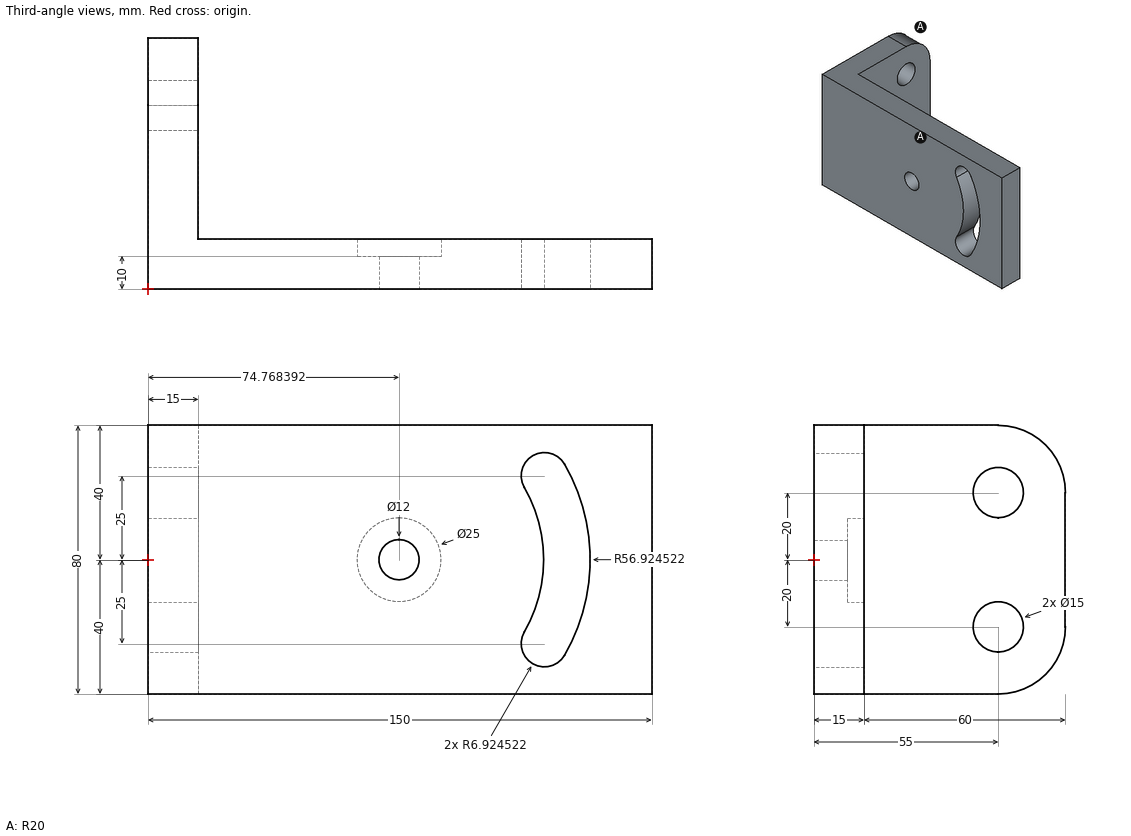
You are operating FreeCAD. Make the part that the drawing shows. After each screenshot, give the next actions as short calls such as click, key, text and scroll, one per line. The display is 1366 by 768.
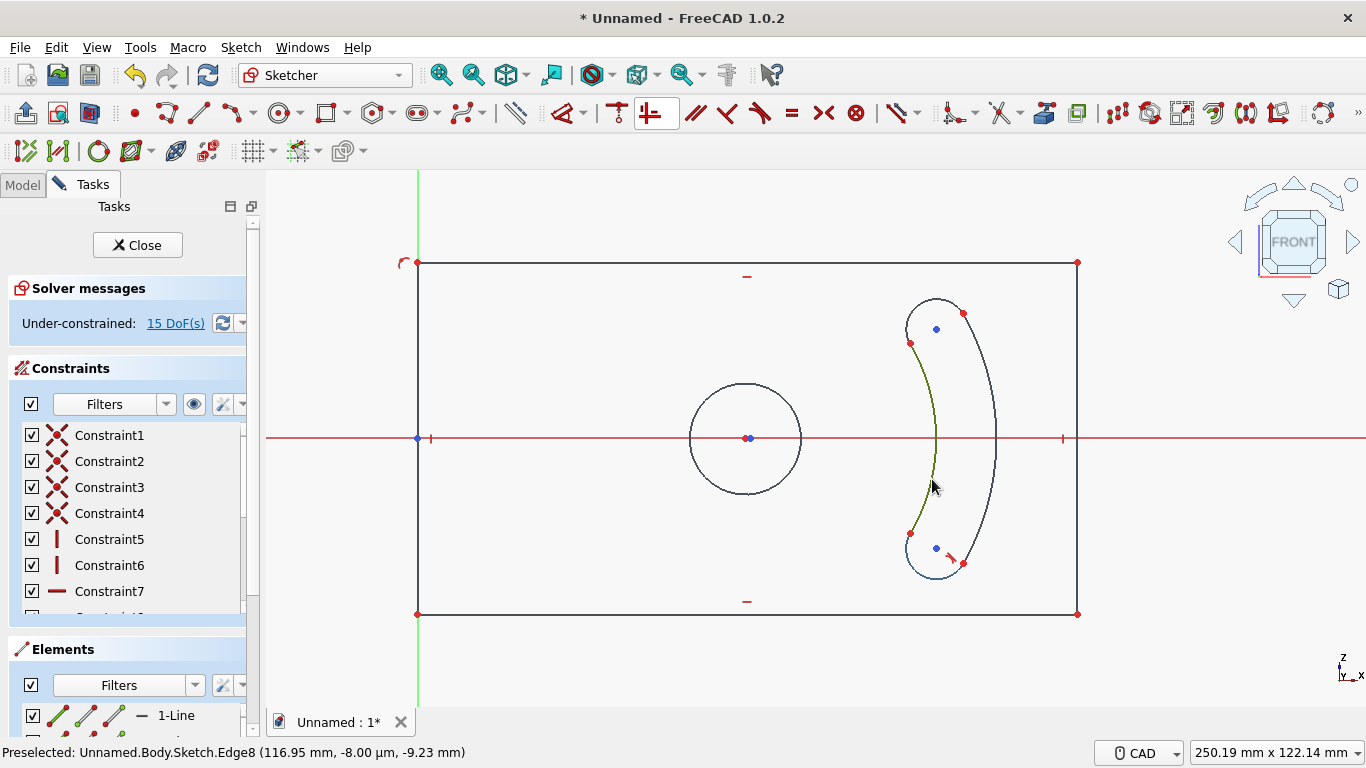
click(760, 114)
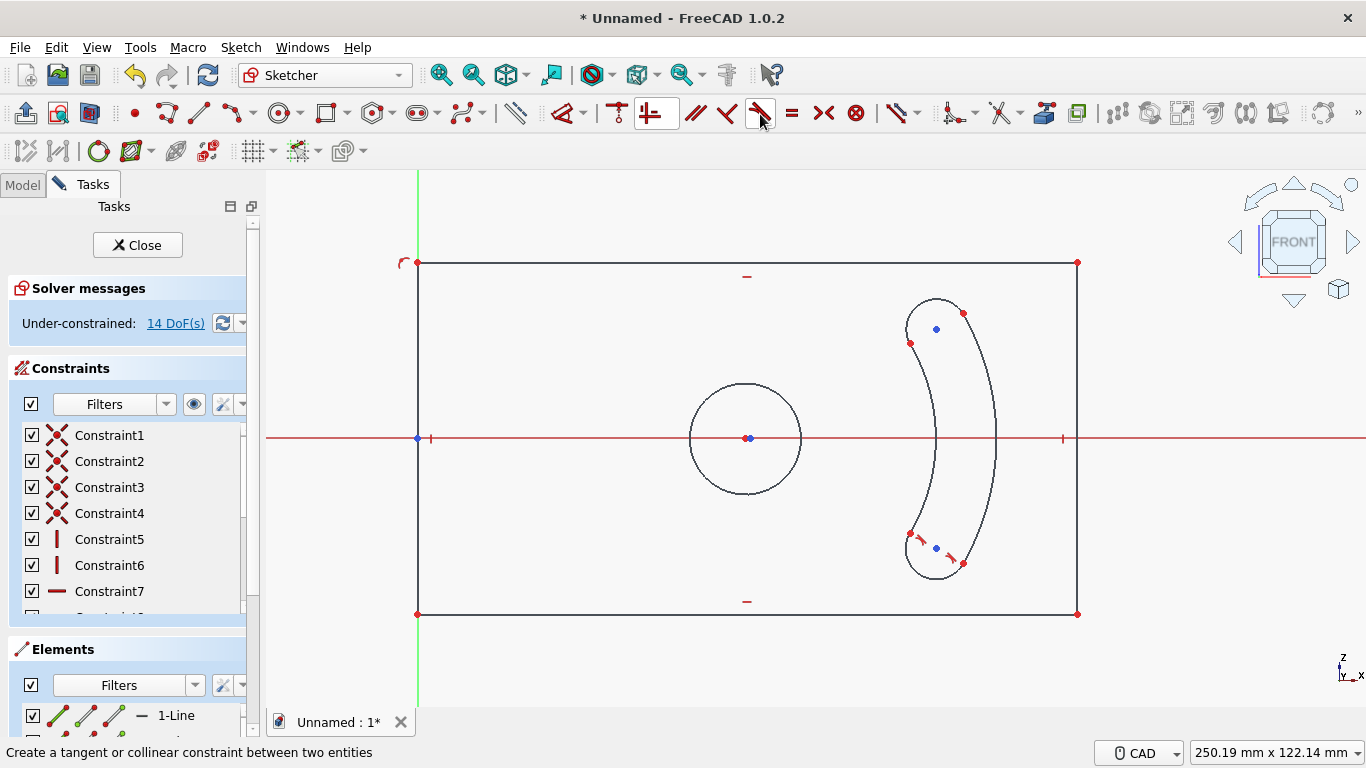
click(991, 491)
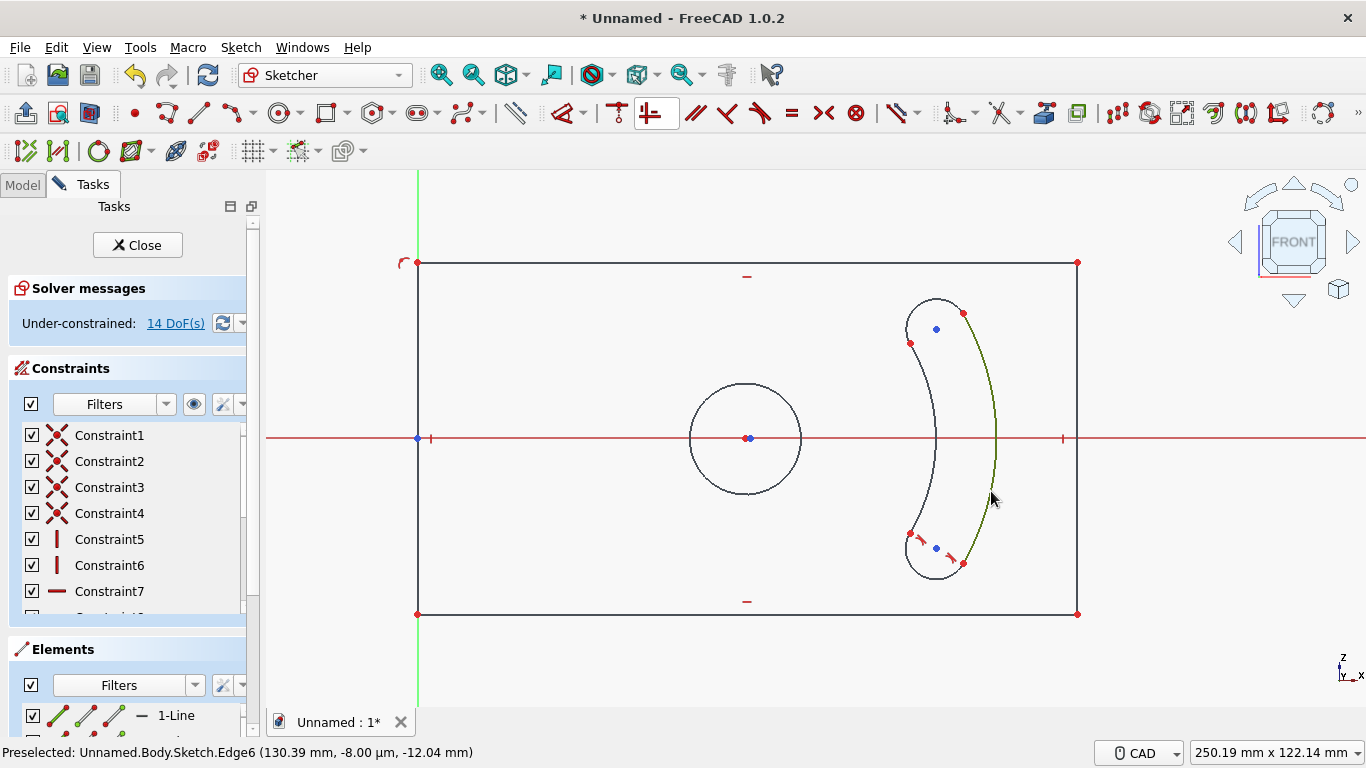
click(940, 299)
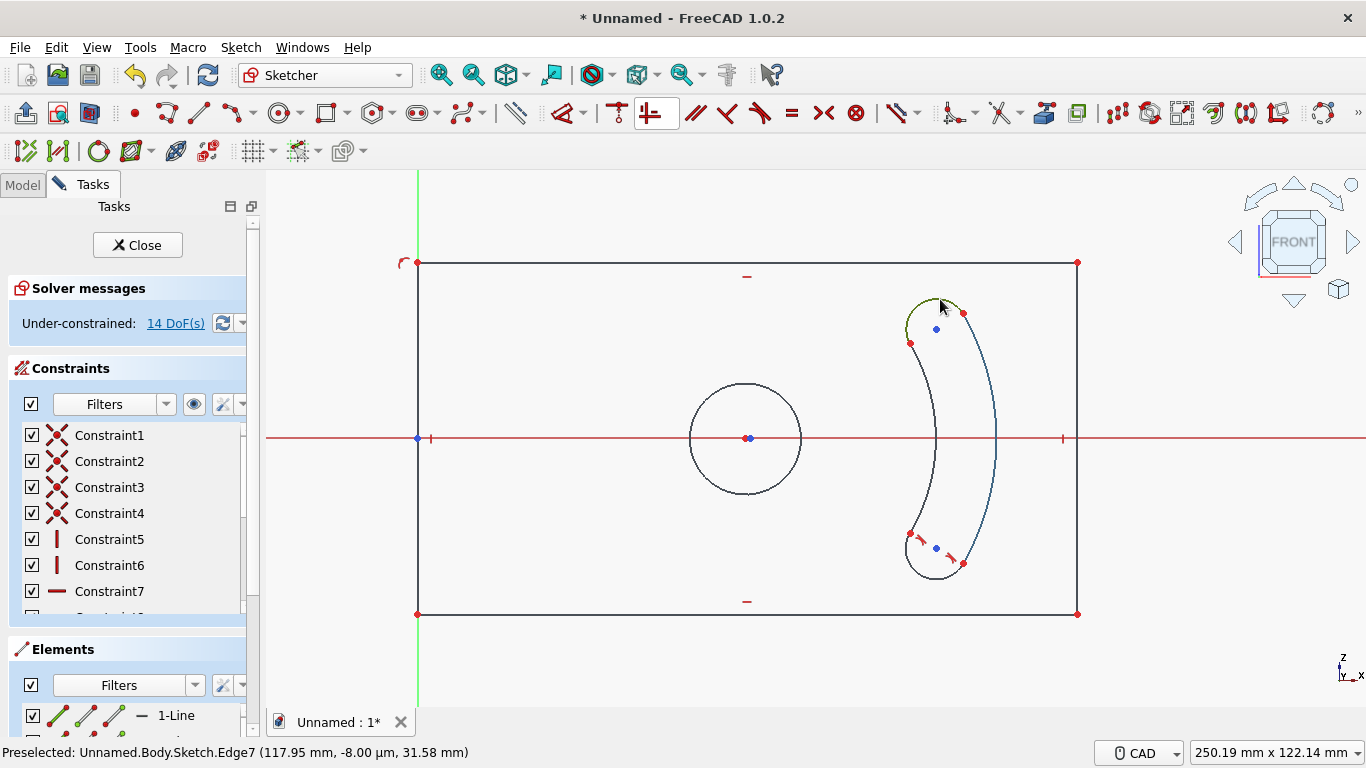
key(t)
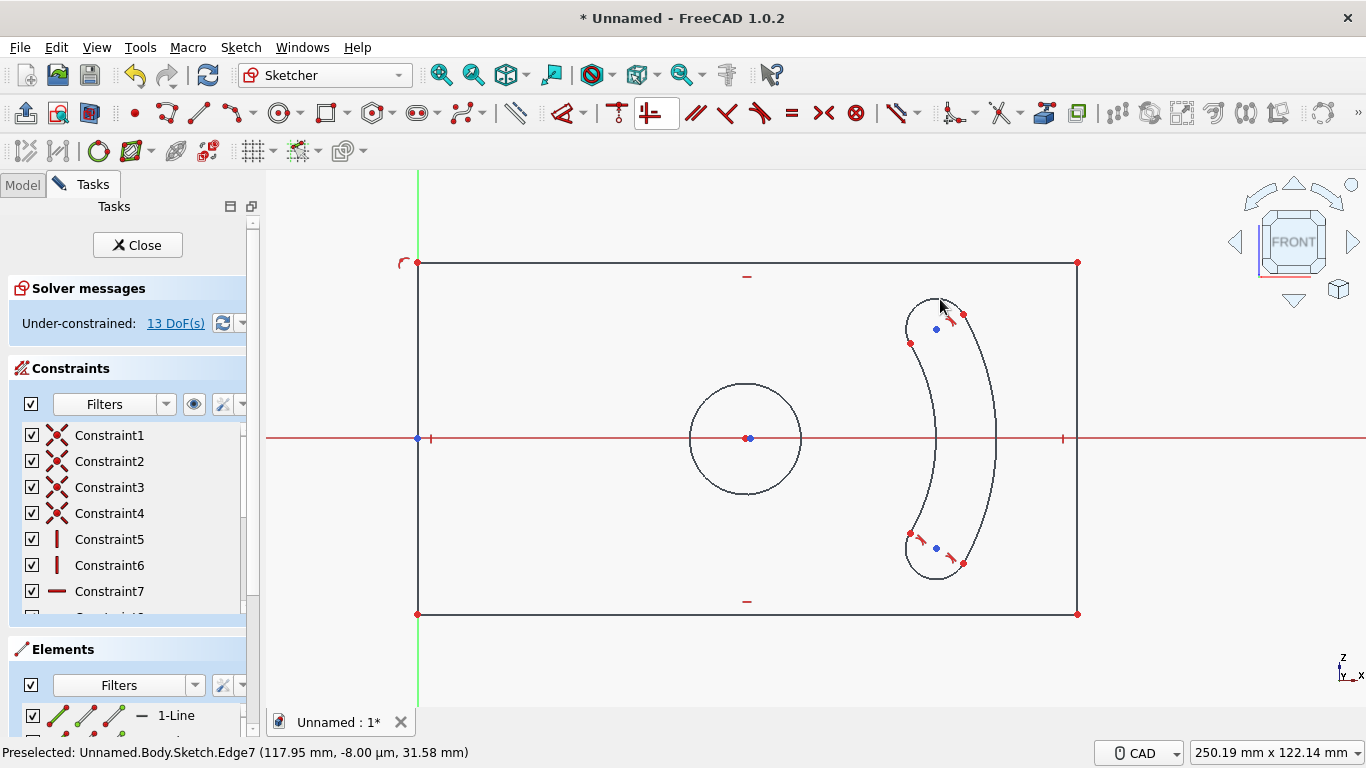
click(940, 299)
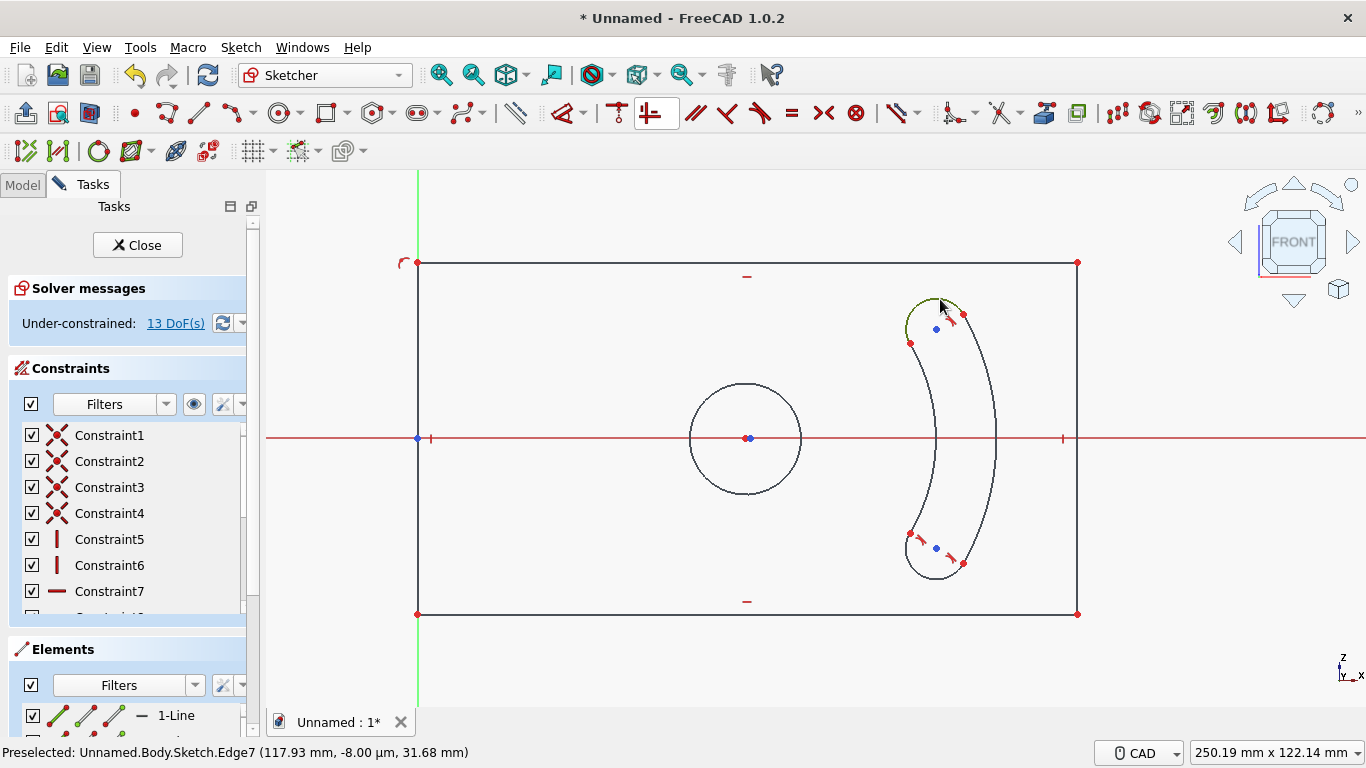
click(932, 478)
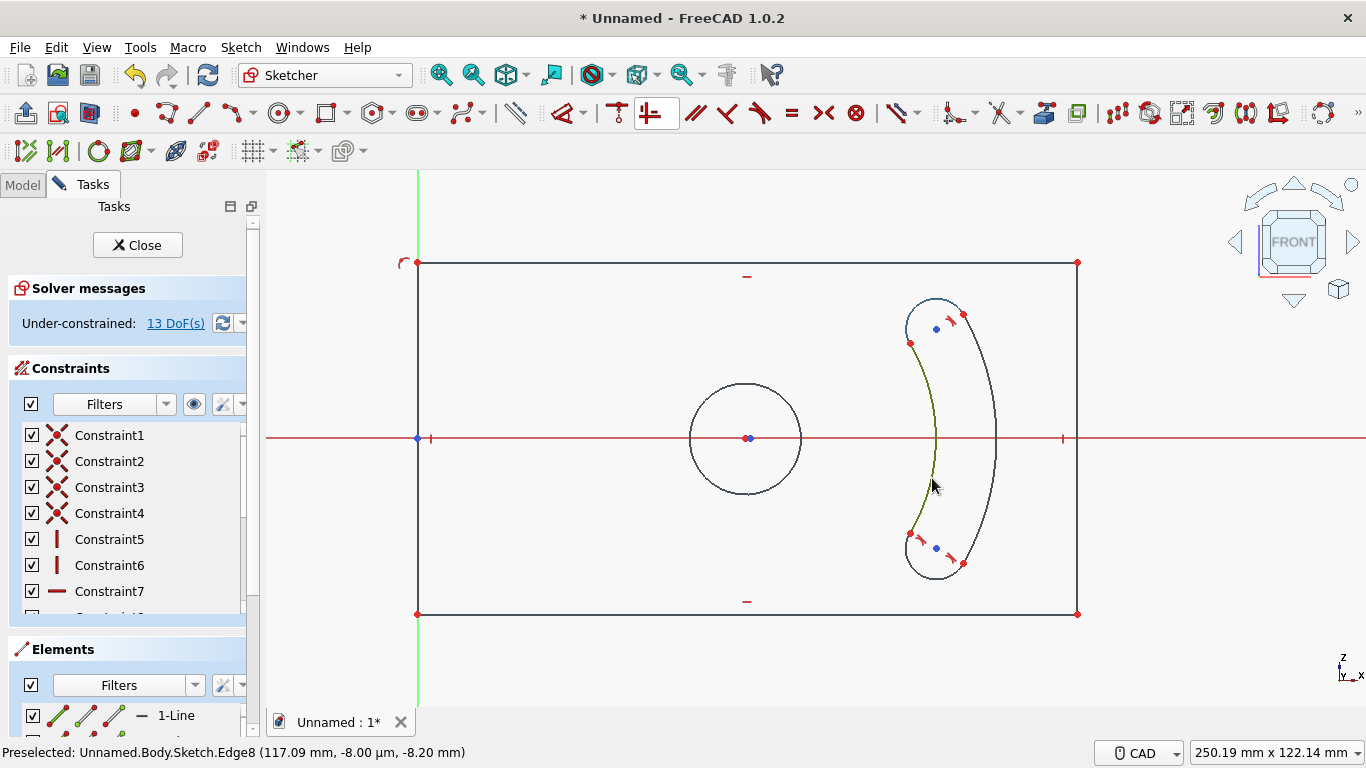
click(760, 114)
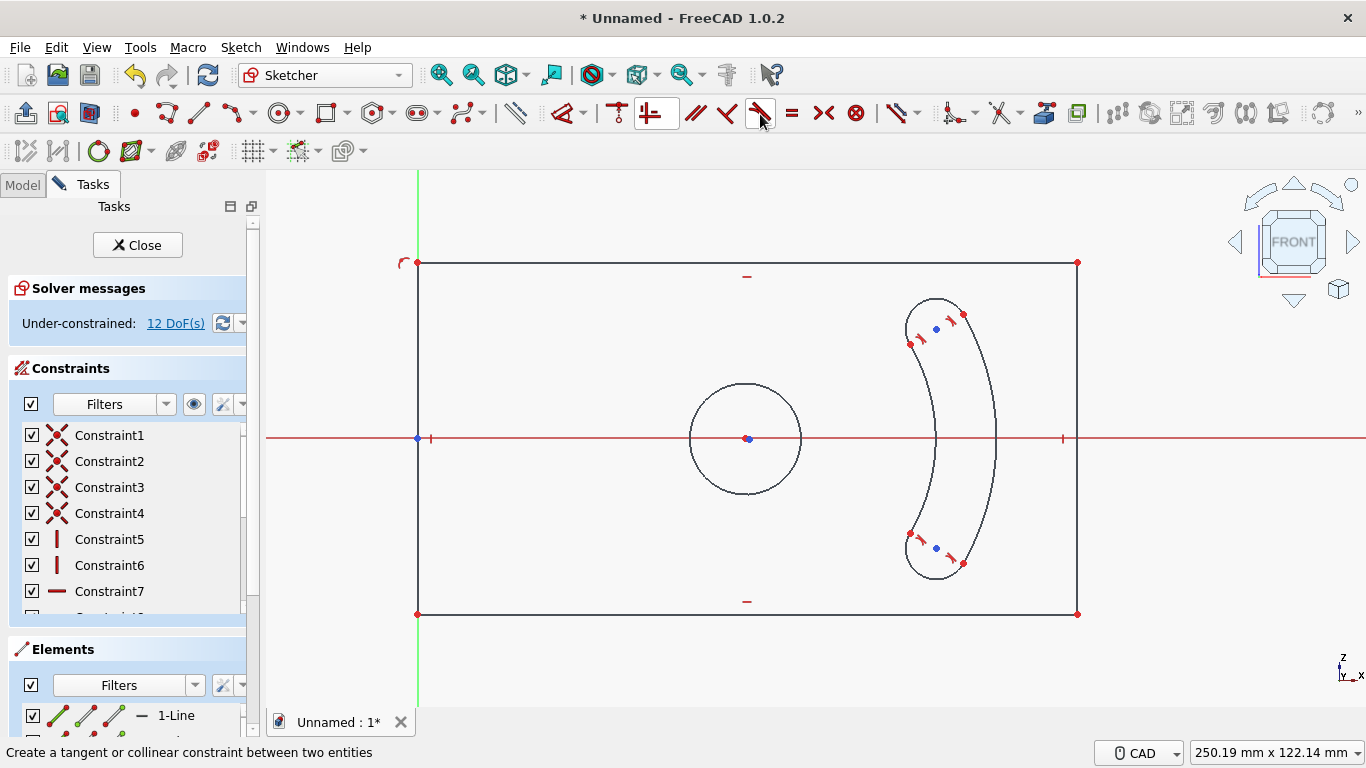
click(785, 400)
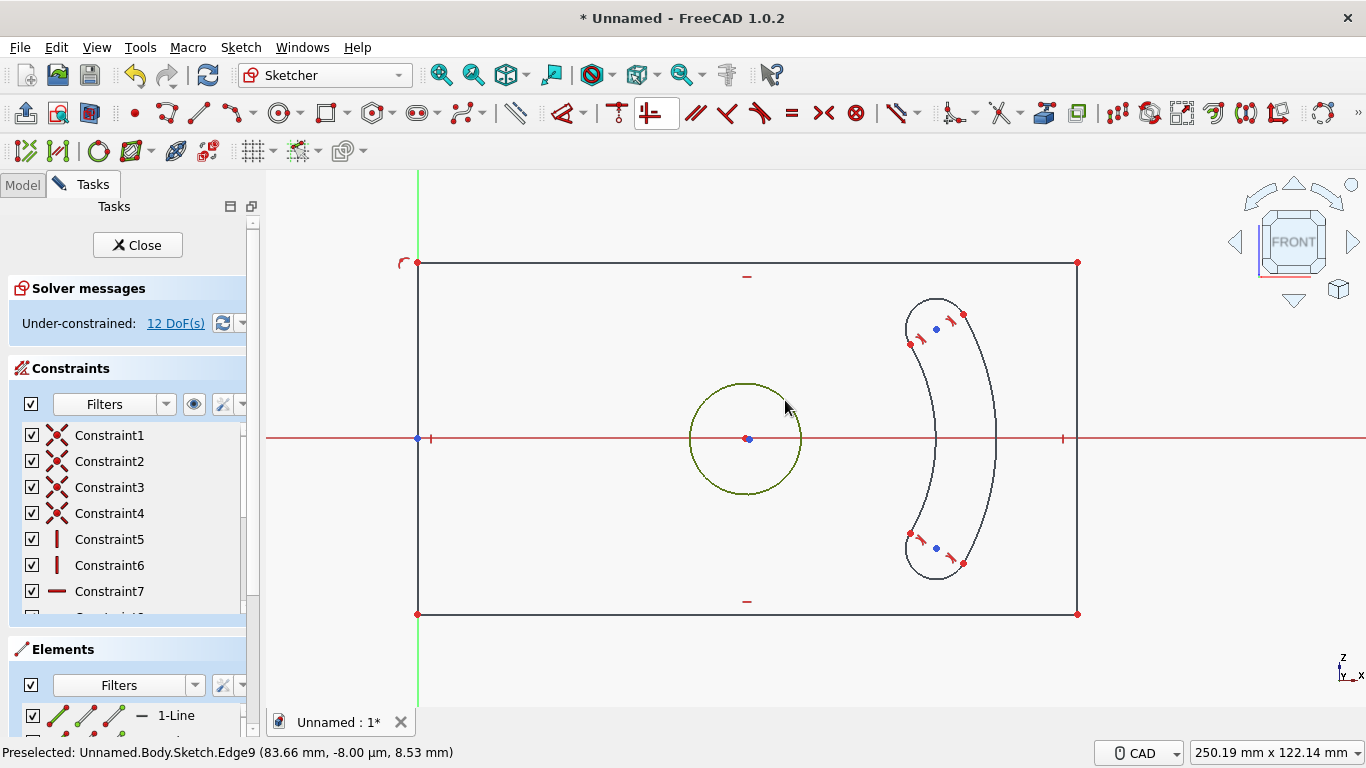
click(931, 478)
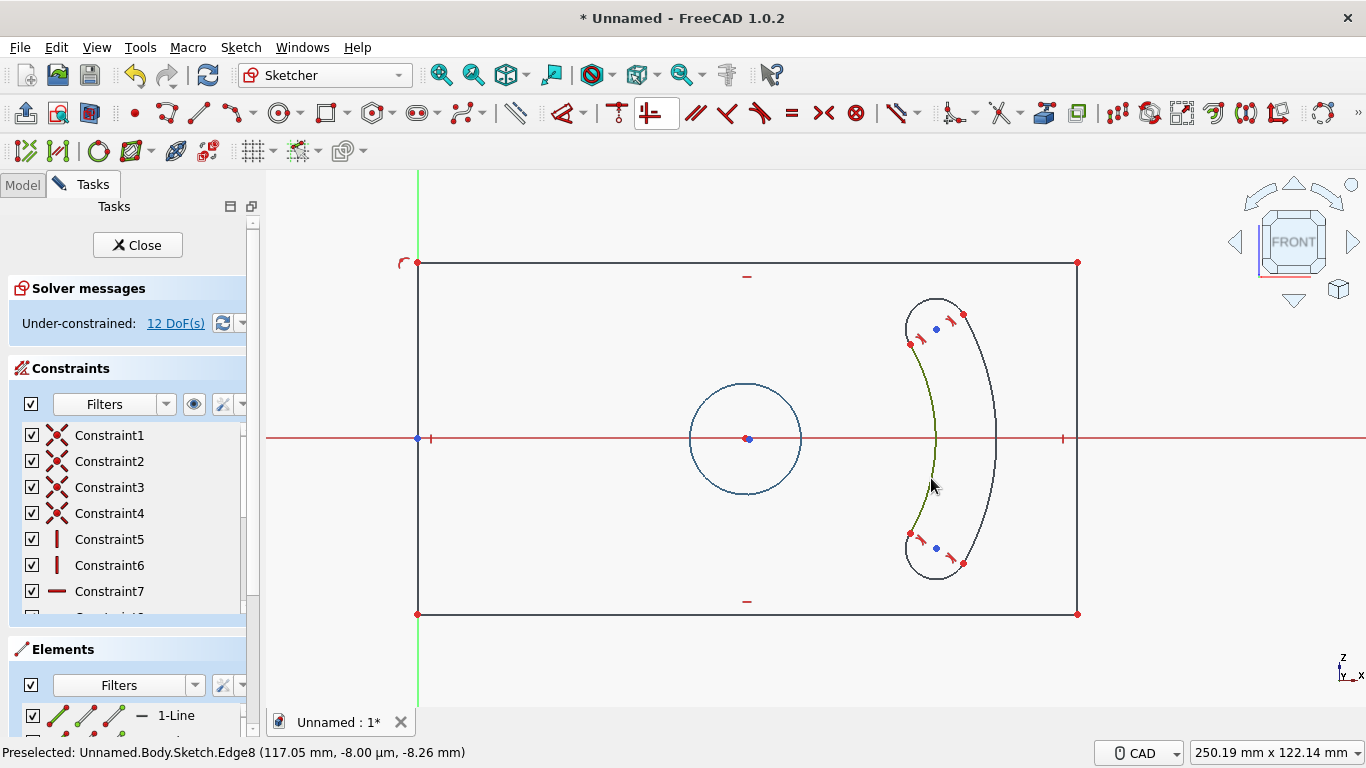
click(618, 114)